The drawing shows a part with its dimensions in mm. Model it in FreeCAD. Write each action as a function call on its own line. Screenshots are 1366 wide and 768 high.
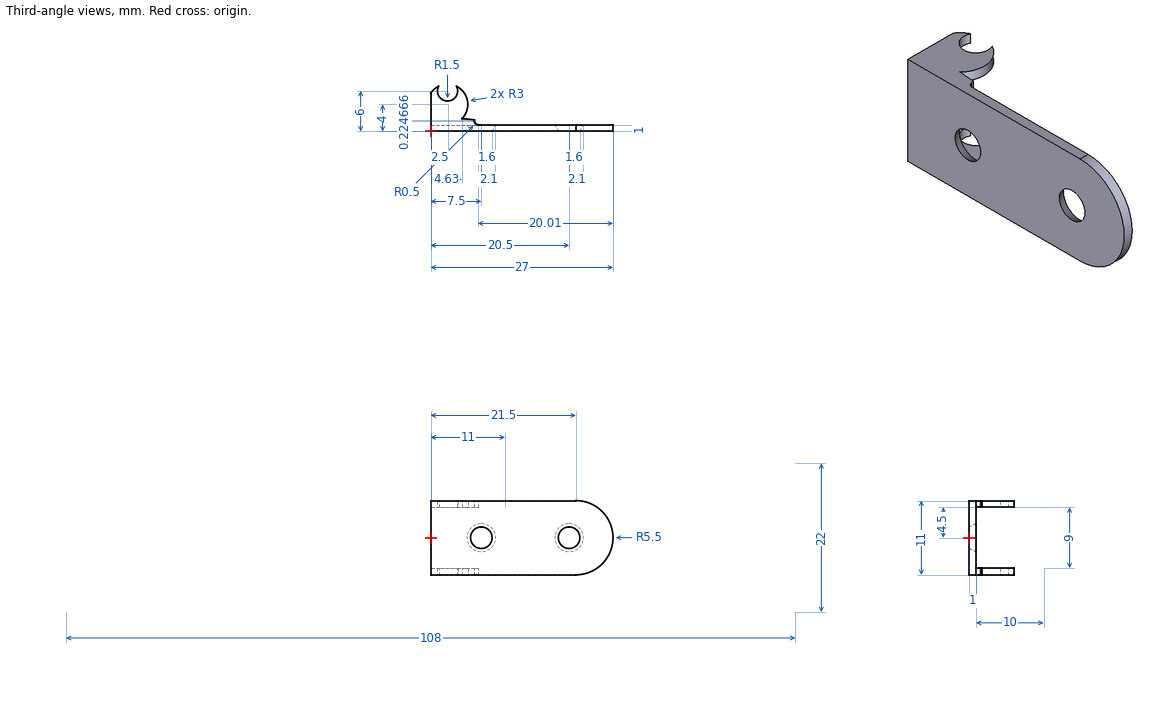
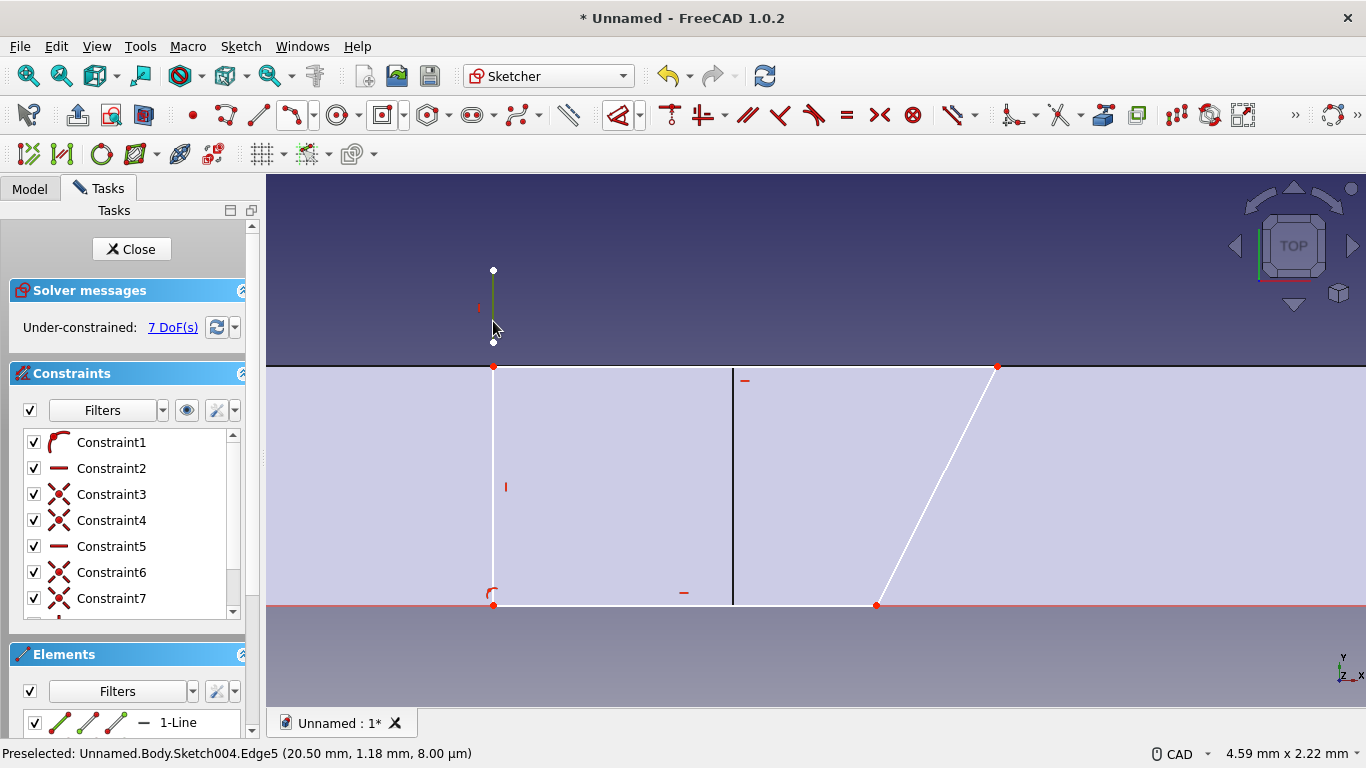
key(g)
key(n)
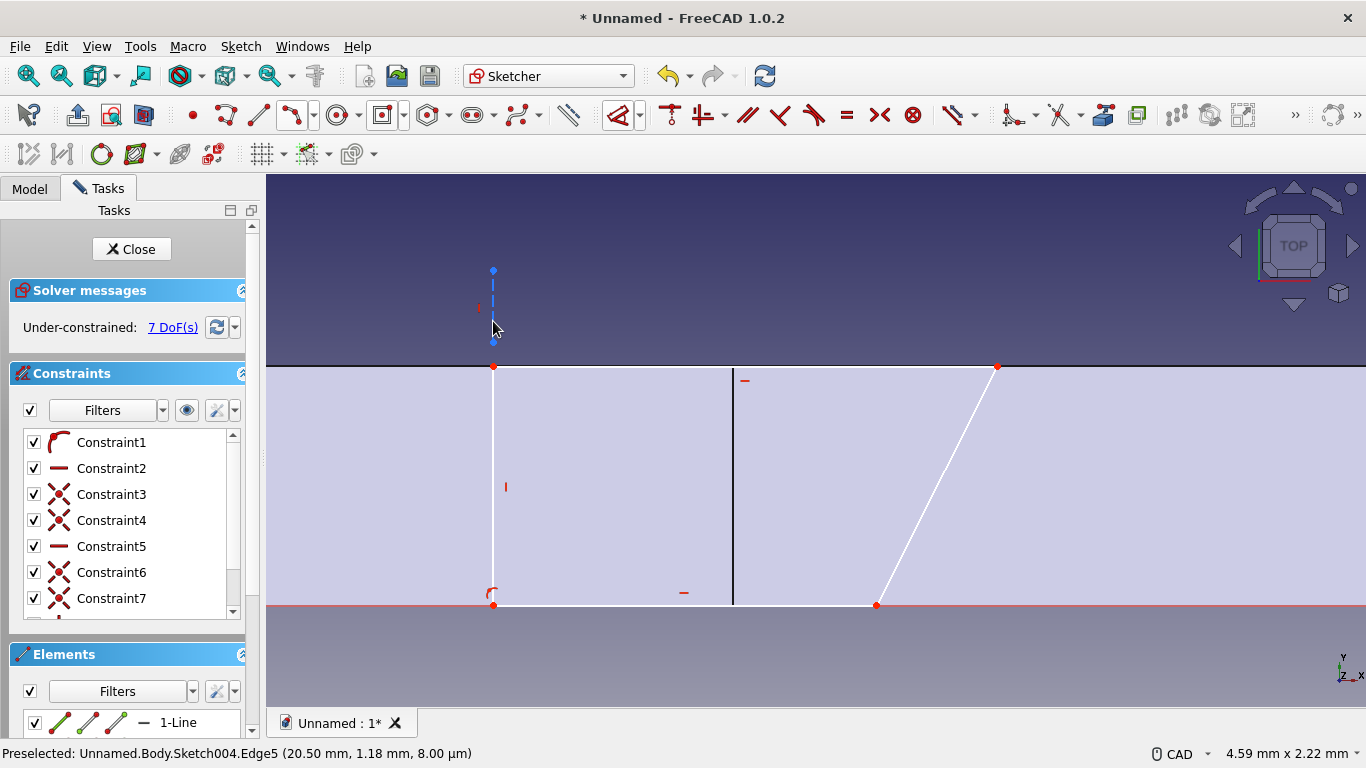
click(493, 439)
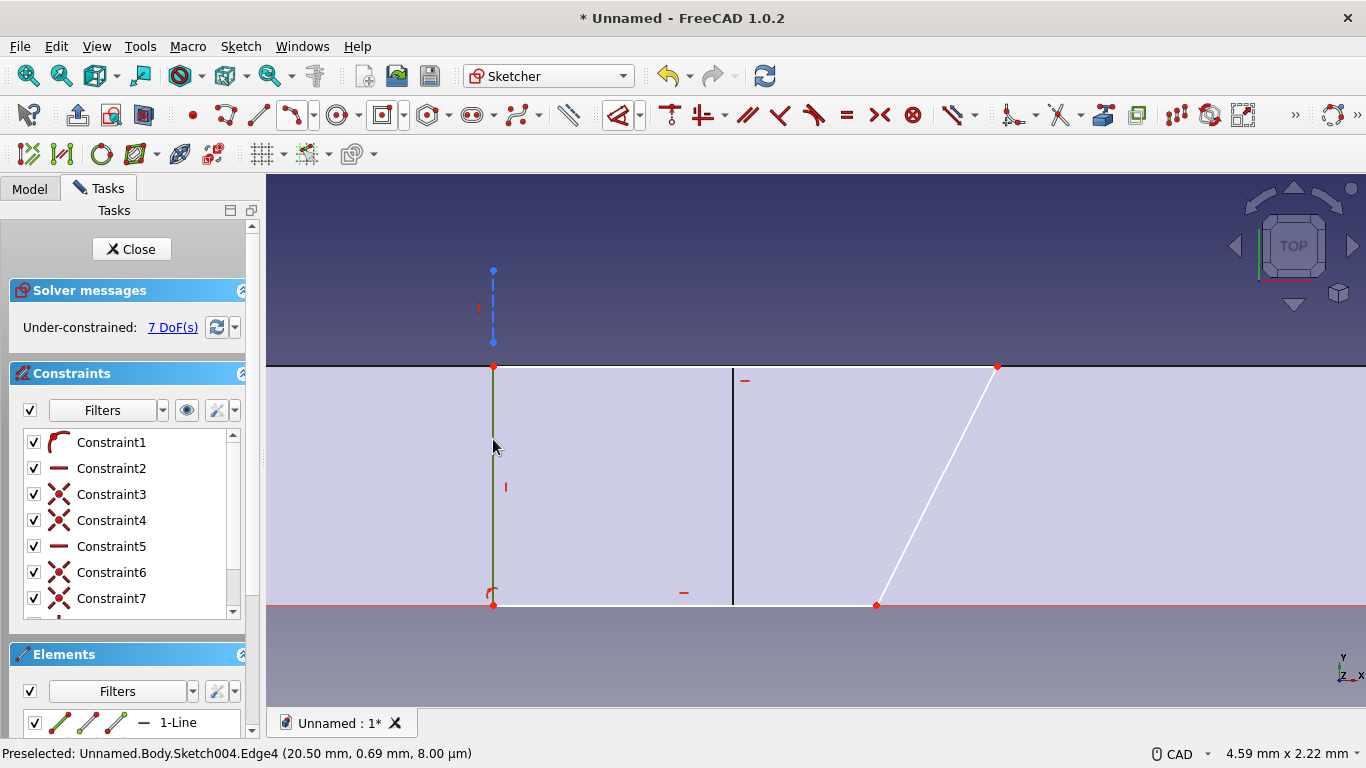
key(i)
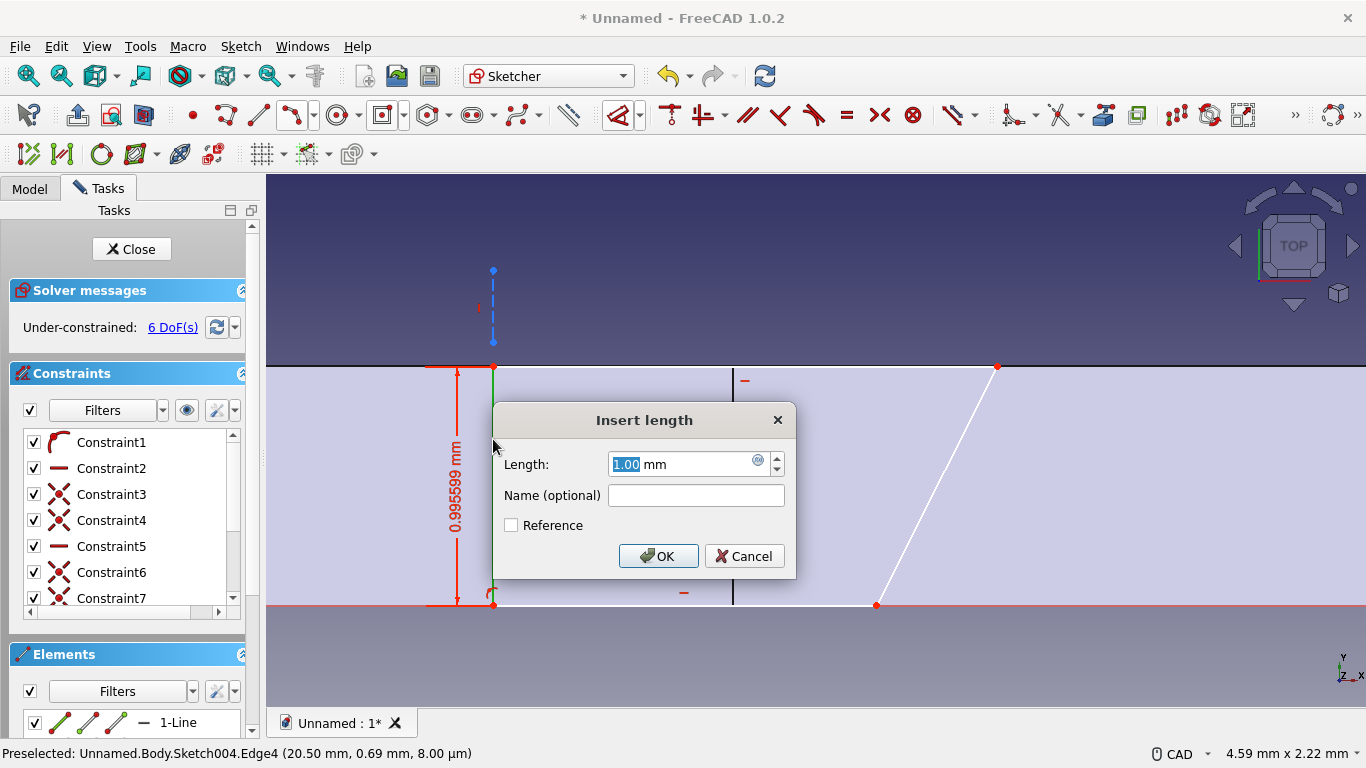
text(1)
key(Return)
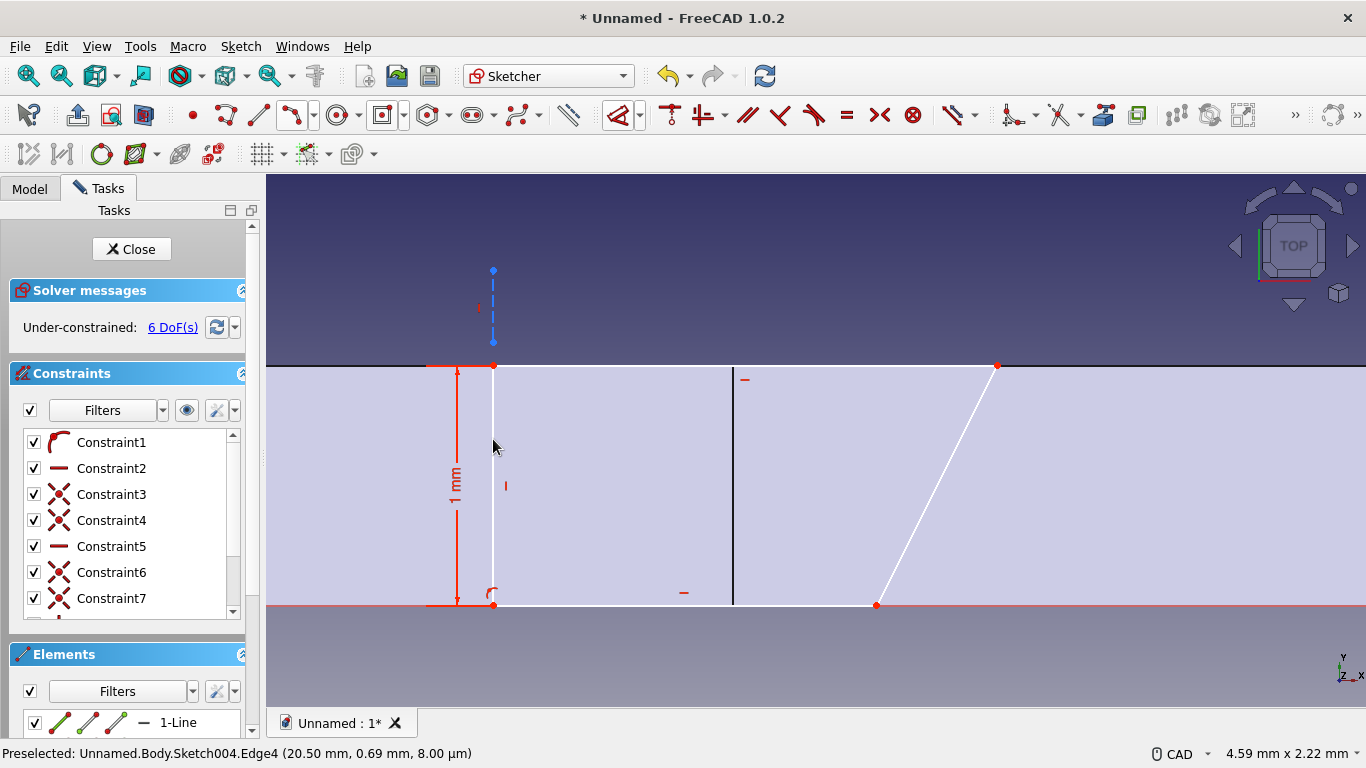
click(608, 606)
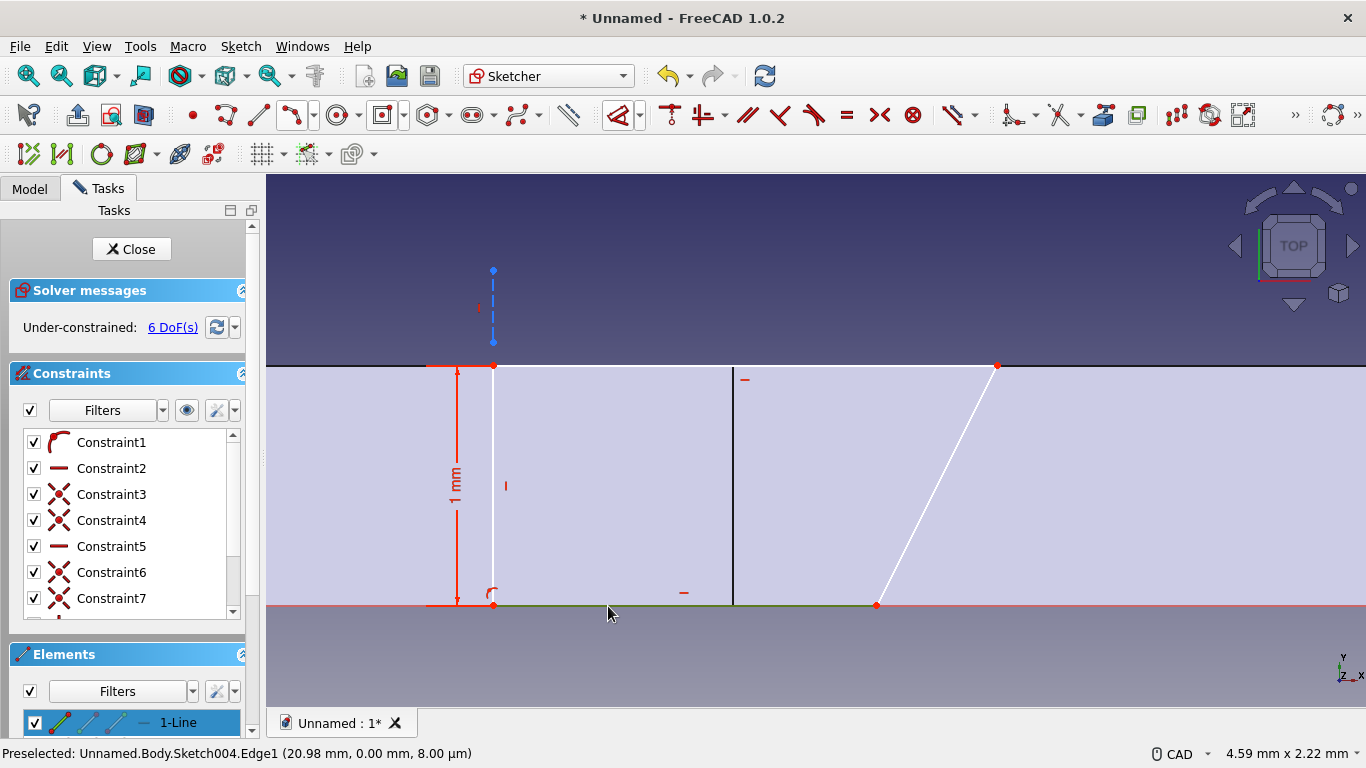
key(l)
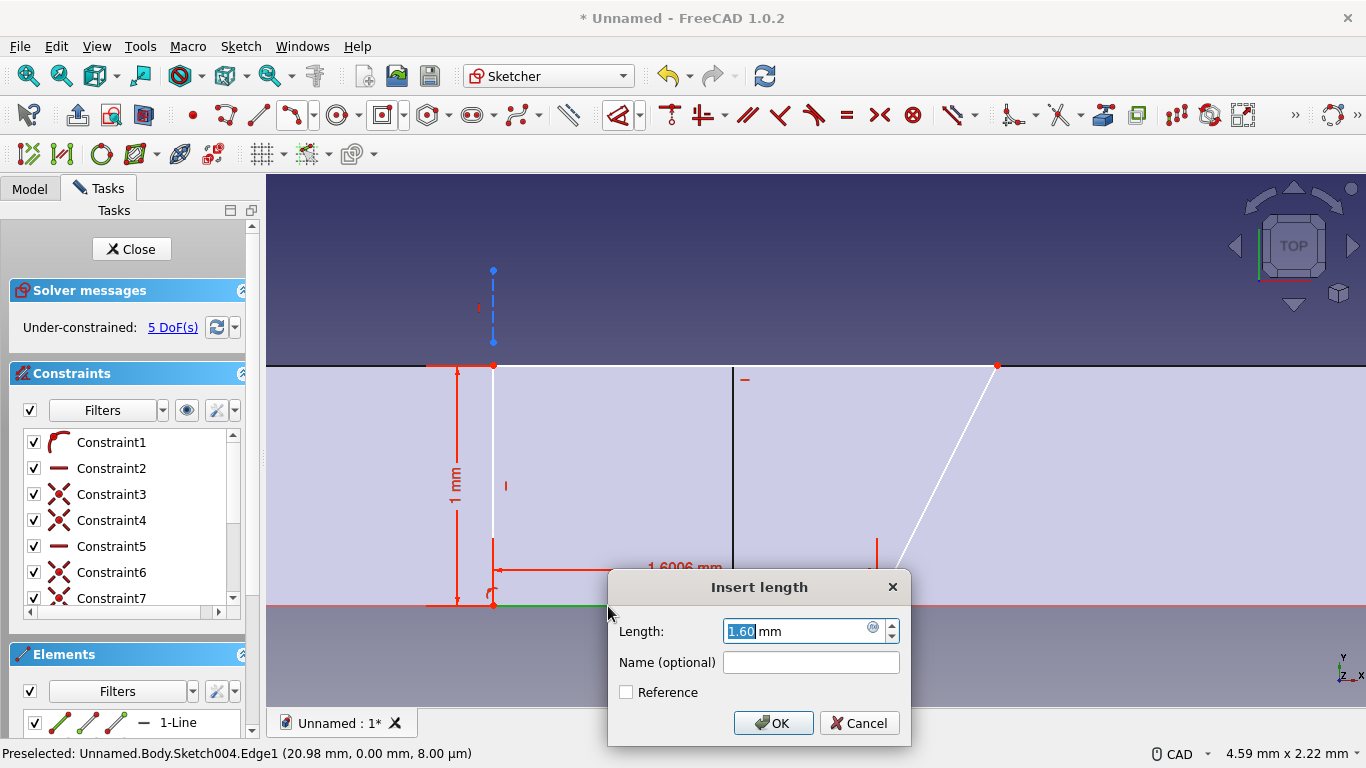
text(1.6)
key(Return)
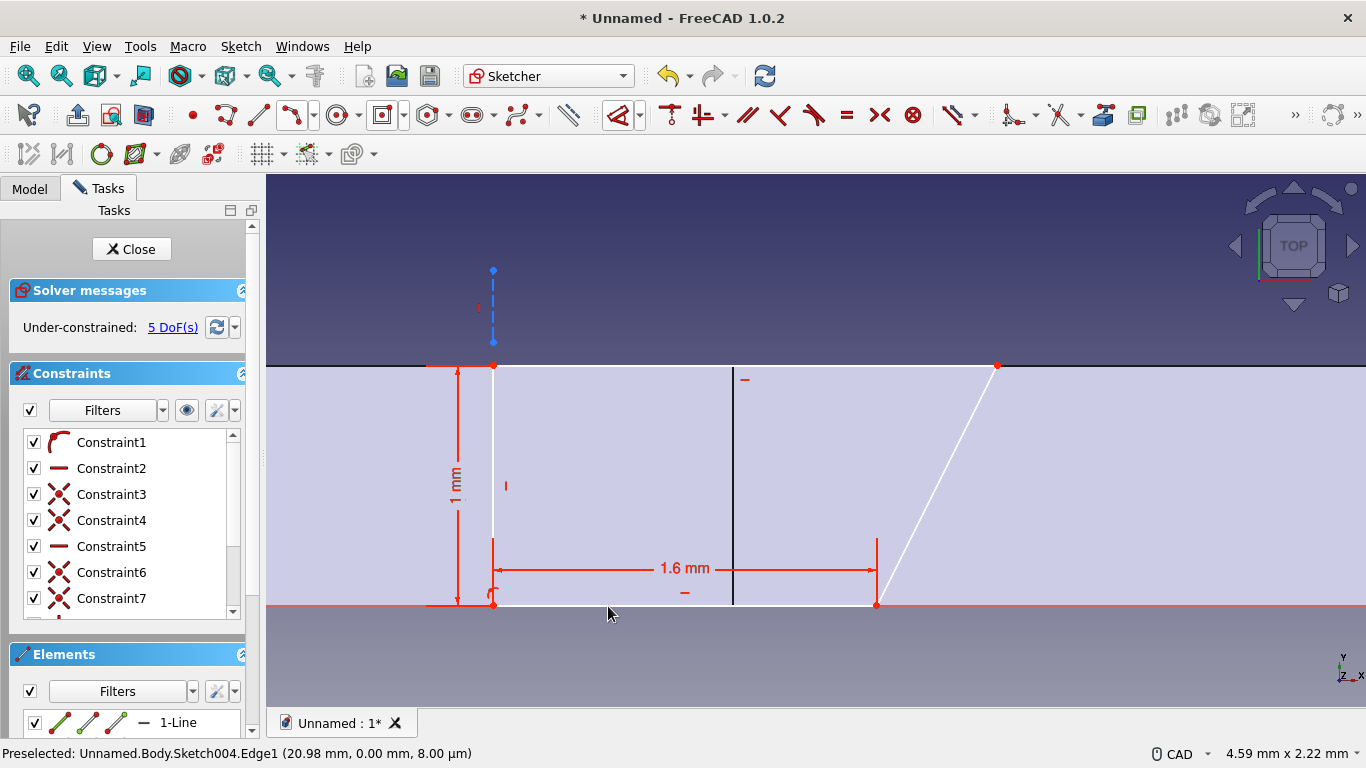
click(846, 366)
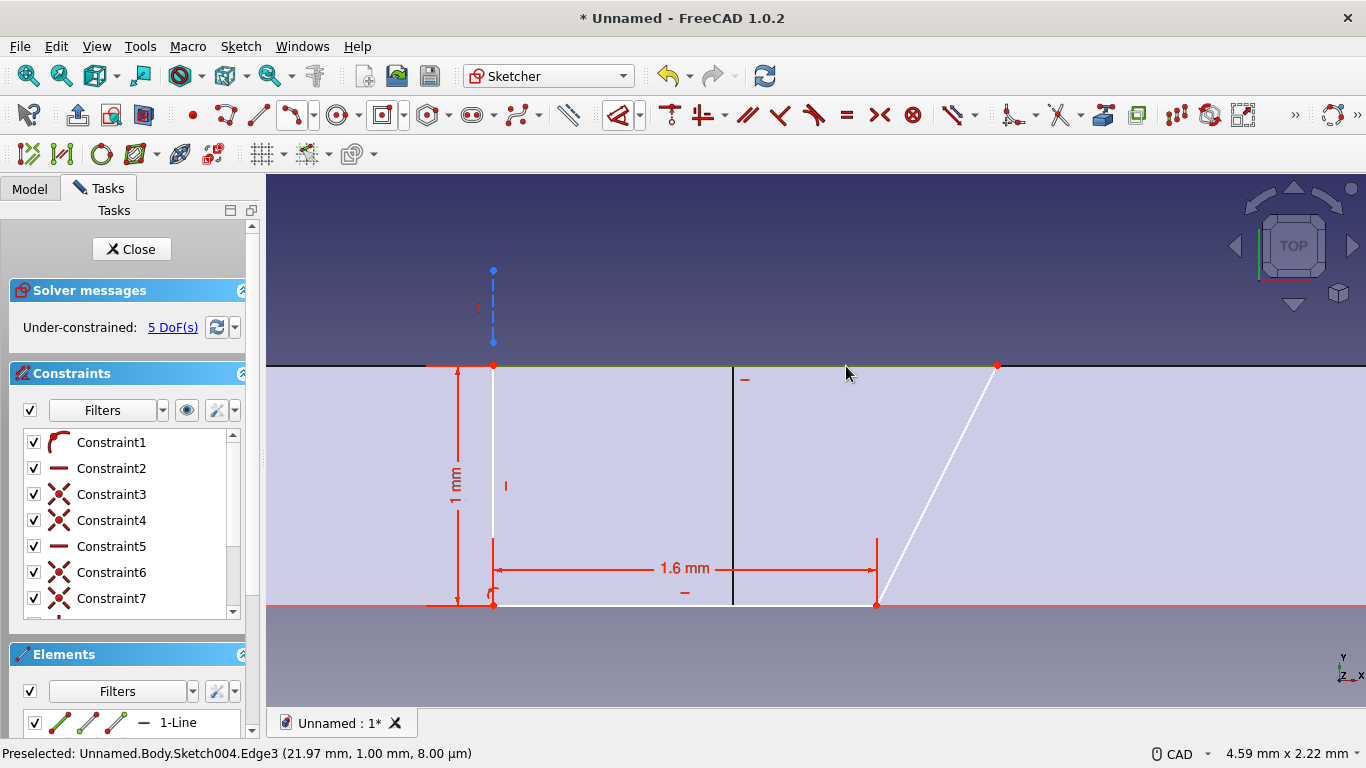
key(l)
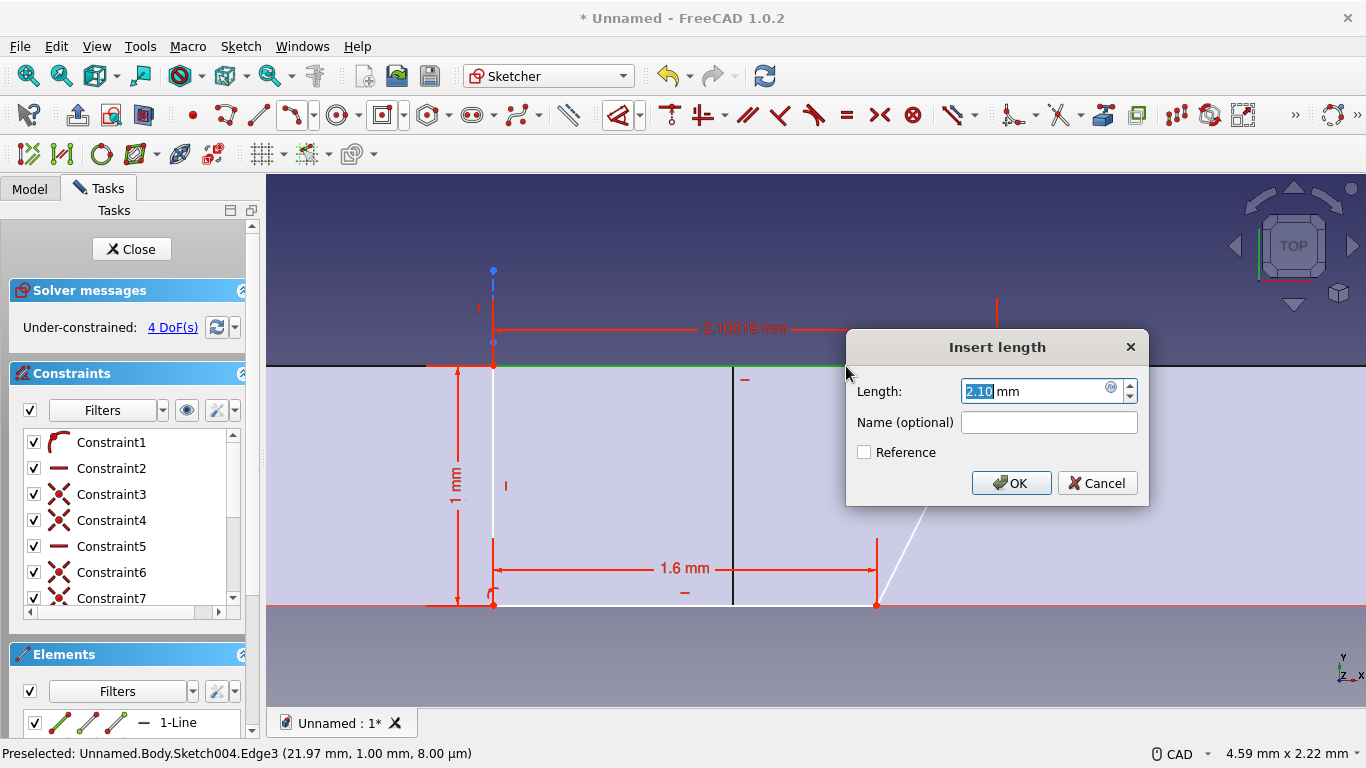
text(2.1)
key(Return)